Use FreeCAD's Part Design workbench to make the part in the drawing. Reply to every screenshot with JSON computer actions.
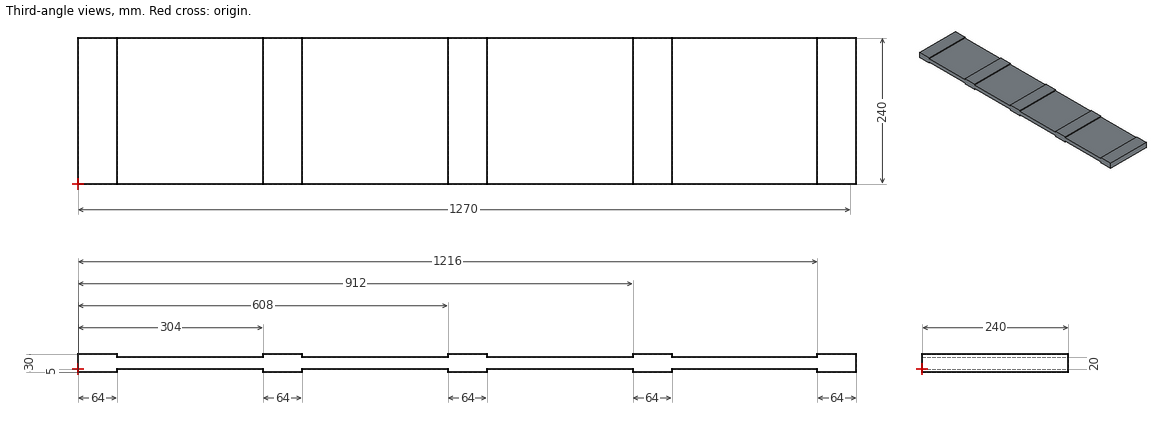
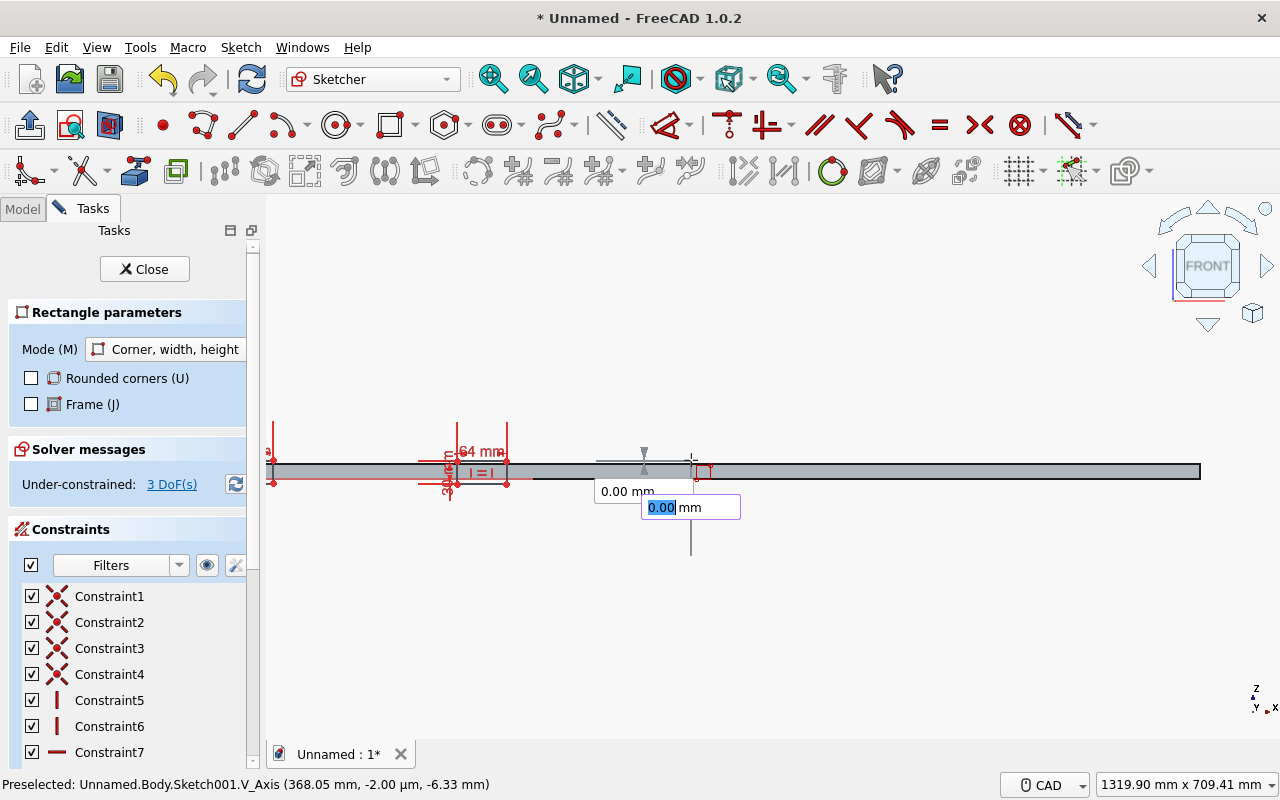
{"action": "scroll", "coordinate": [740, 483], "scroll_direction": "up", "scroll_amount": 8}
{"action": "mouse_move", "coordinate": [739, 482]}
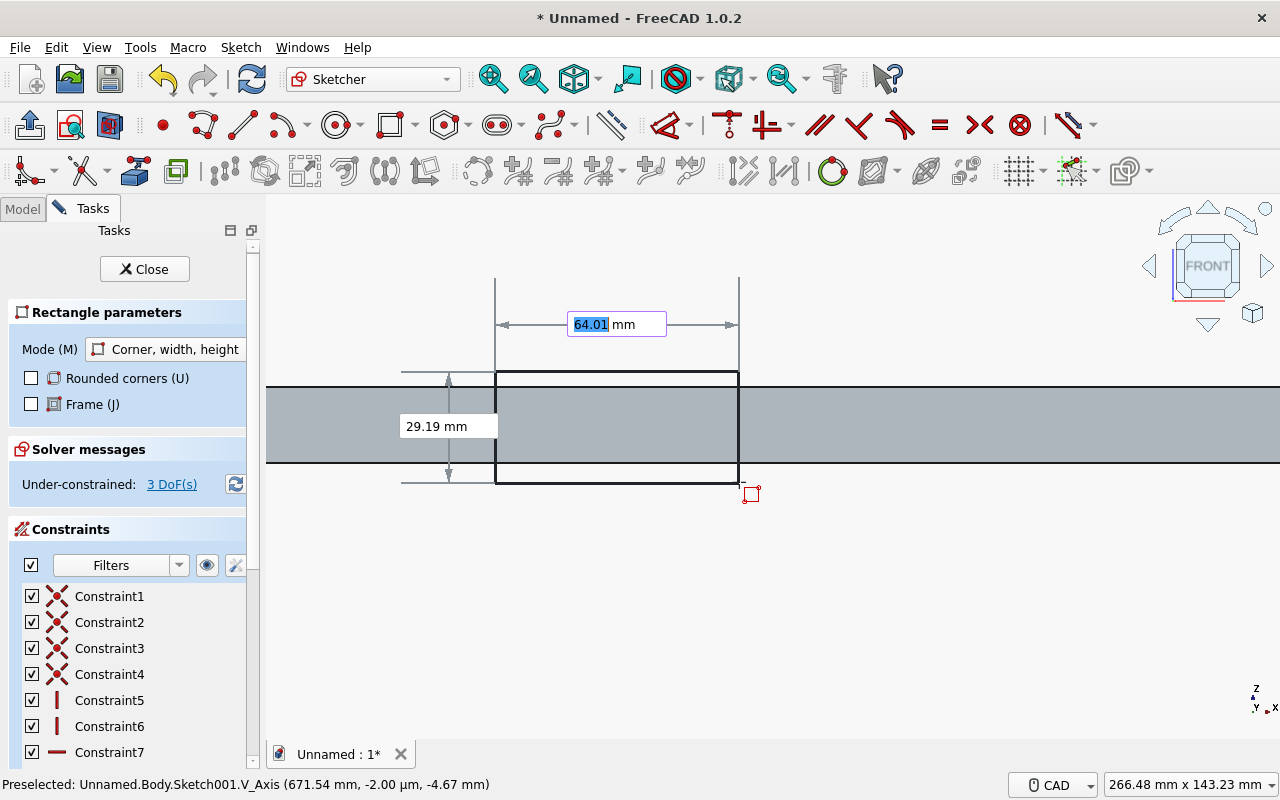
{"action": "type", "text": "64"}
{"action": "key", "text": "Tab"}
{"action": "type", "text": "30"}
{"action": "key", "text": "Return"}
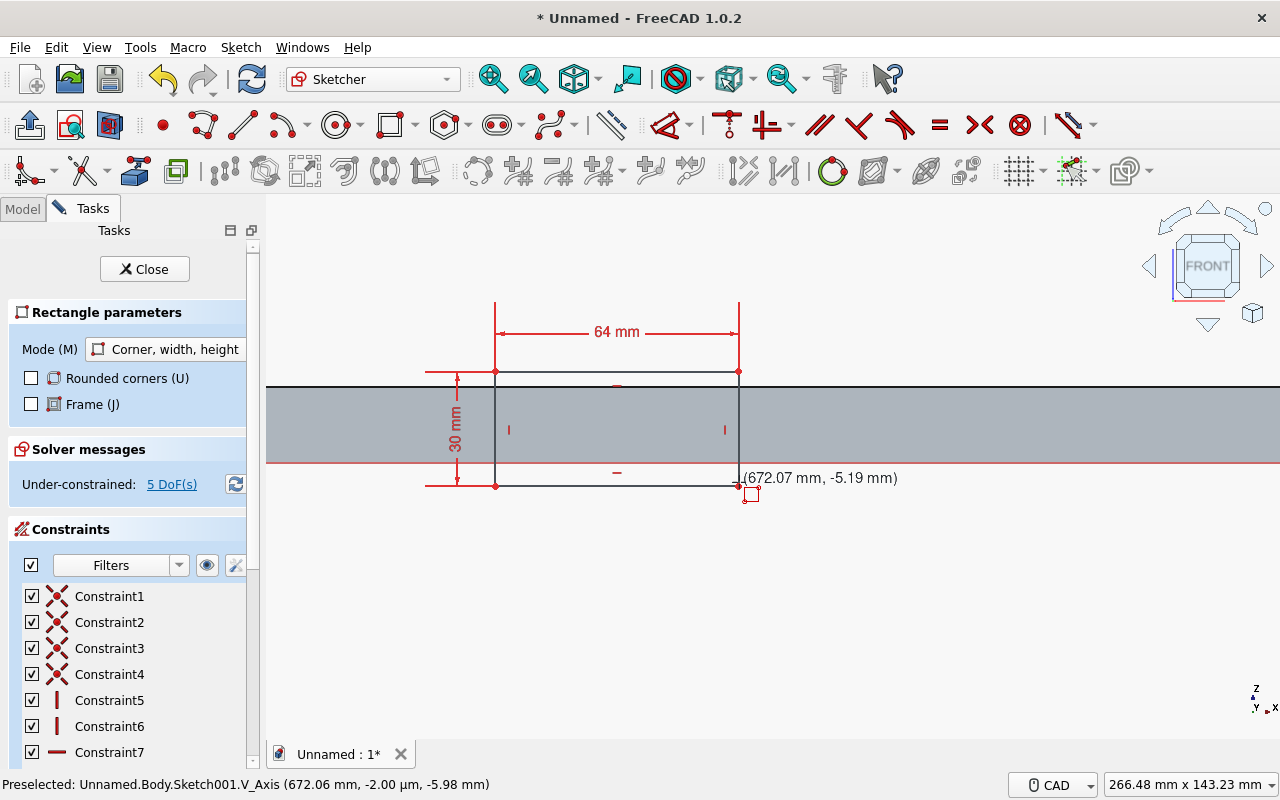
{"action": "scroll", "coordinate": [715, 472], "scroll_direction": "down", "scroll_amount": 11}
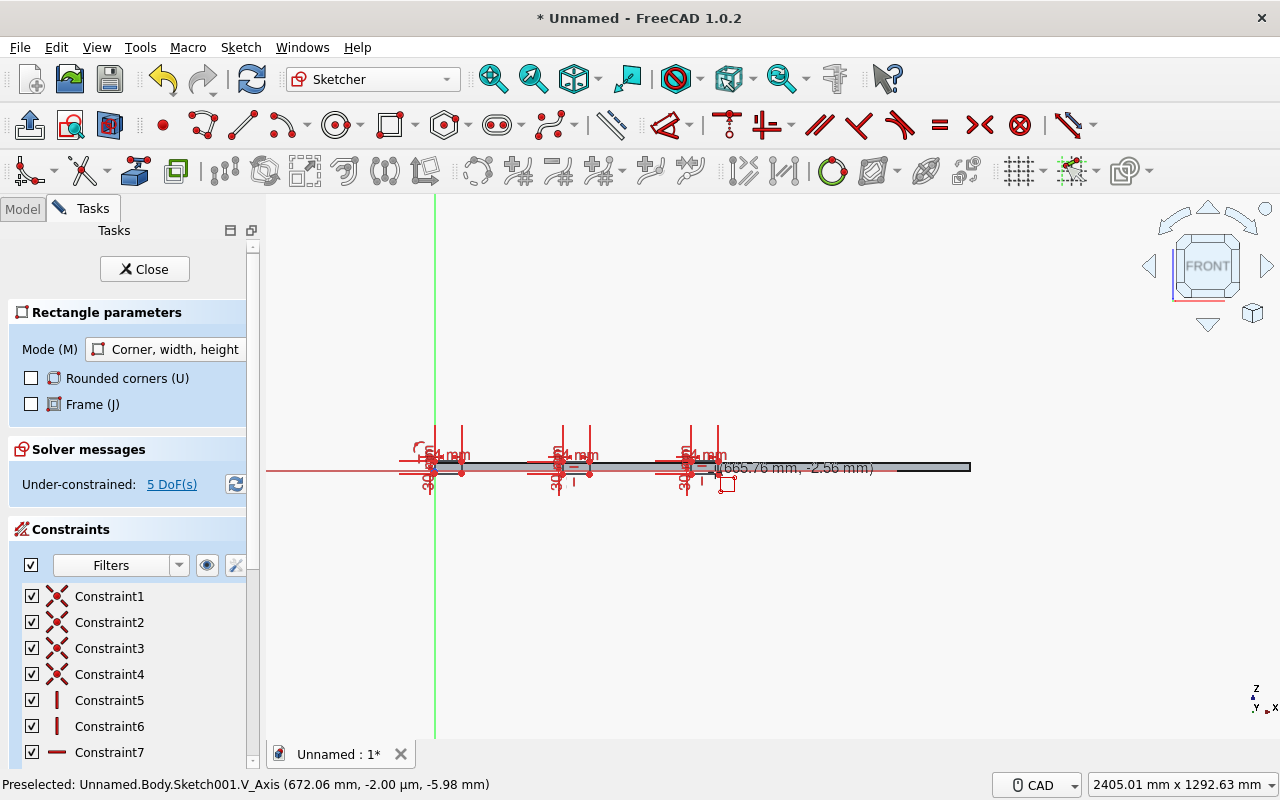
{"action": "scroll", "coordinate": [819, 461], "scroll_direction": "up", "scroll_amount": 3}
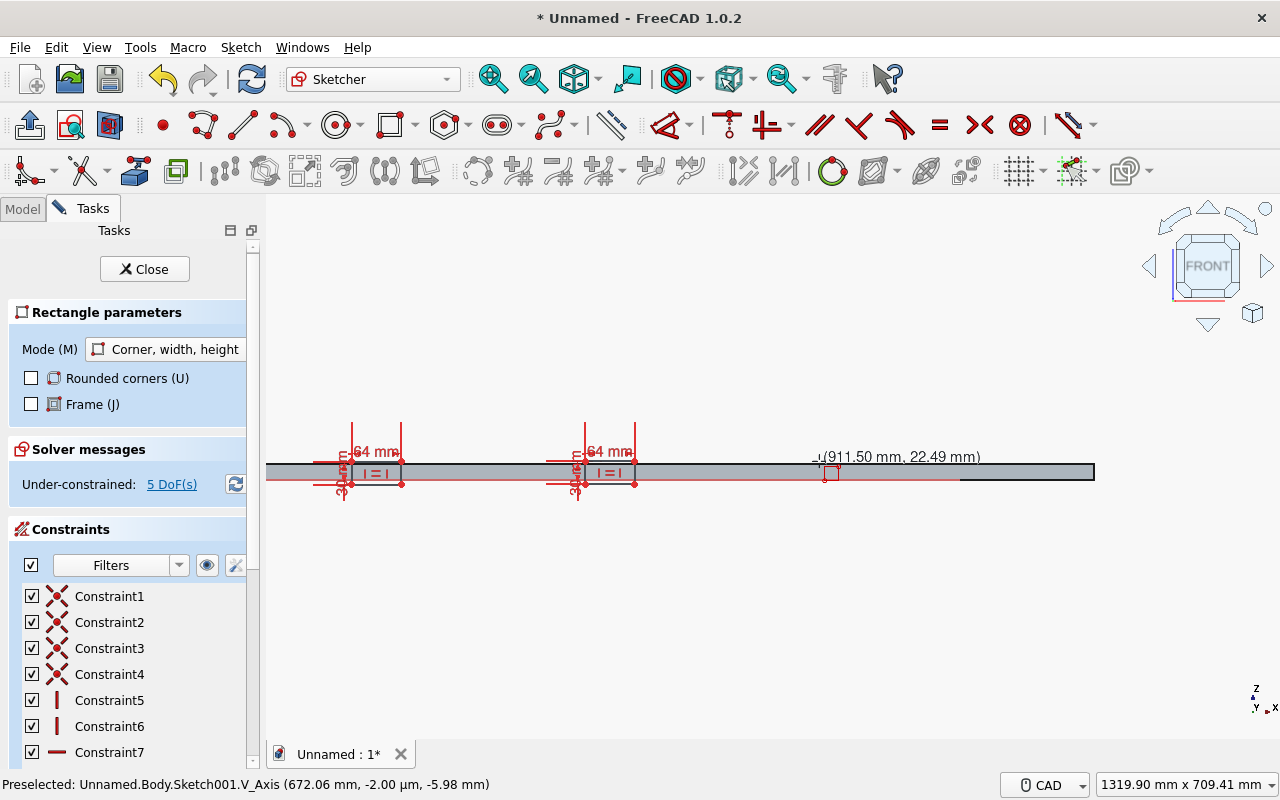
{"action": "left_click", "coordinate": [819, 460]}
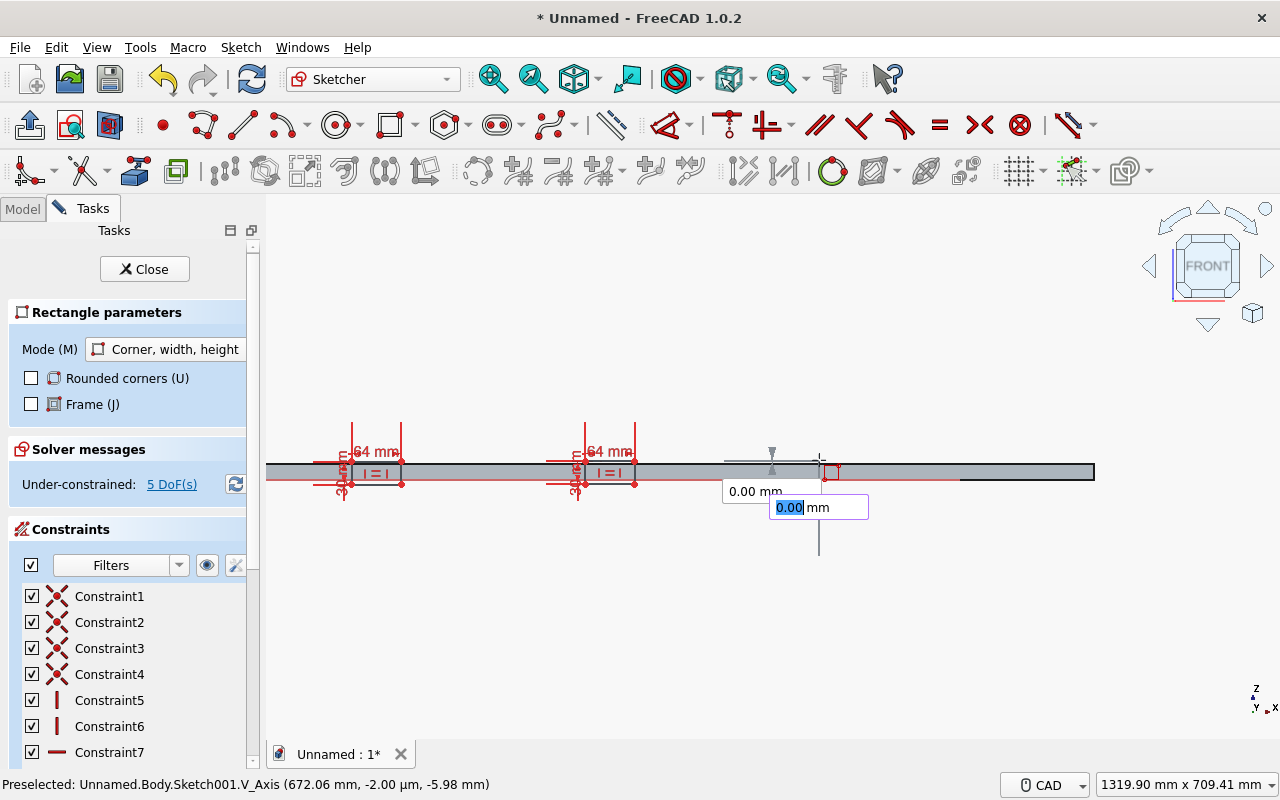
{"action": "scroll", "coordinate": [868, 484], "scroll_direction": "up", "scroll_amount": 8}
{"action": "mouse_move", "coordinate": [866, 480]}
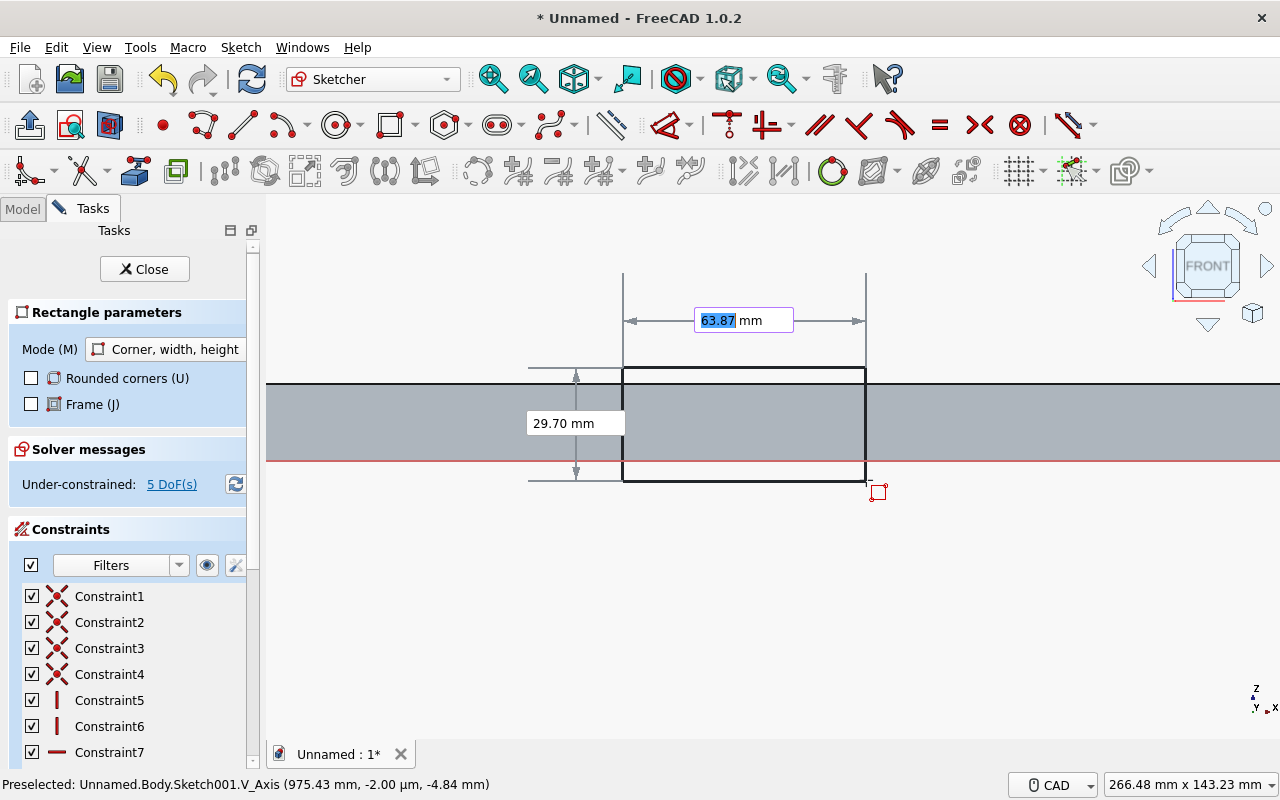
{"action": "type", "text": "64"}
{"action": "key", "text": "Tab"}
{"action": "type", "text": "30"}
{"action": "key", "text": "Return"}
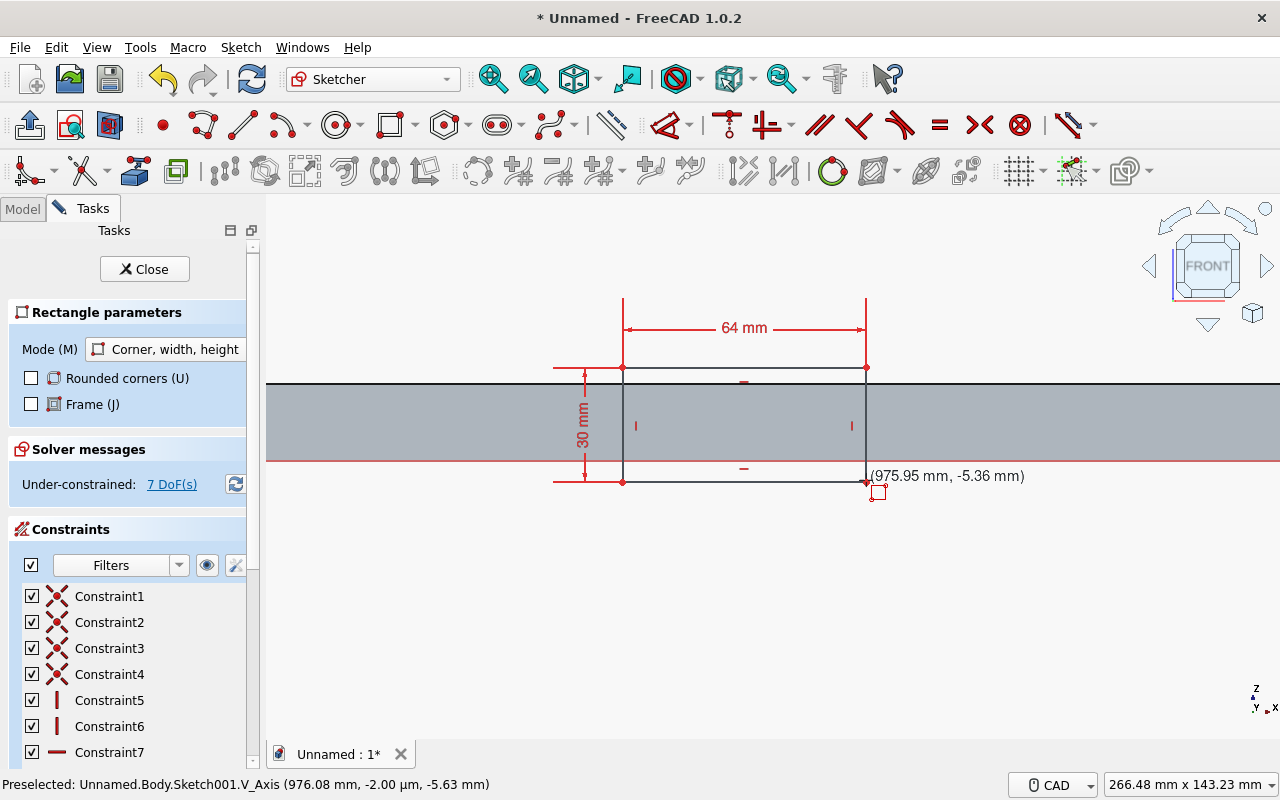
{"action": "scroll", "coordinate": [844, 472], "scroll_direction": "down", "scroll_amount": 11}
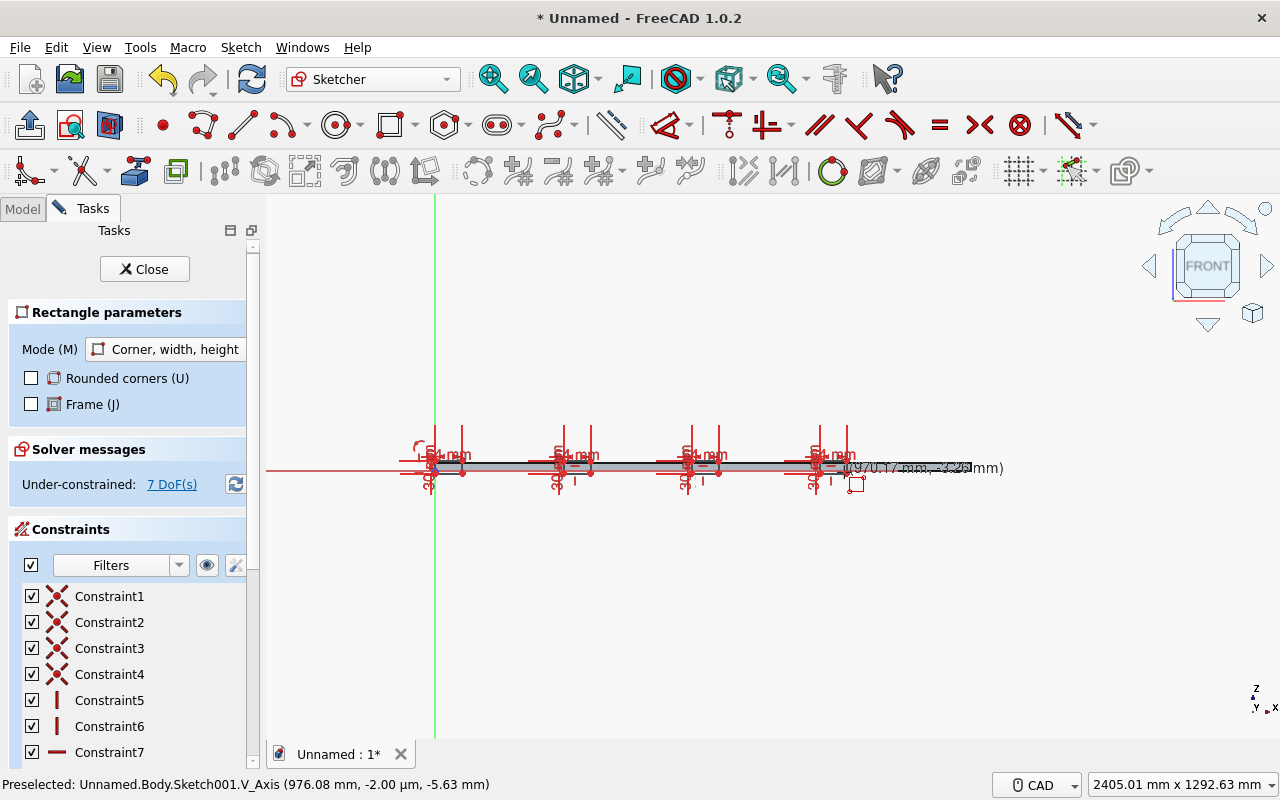
{"action": "scroll", "coordinate": [948, 461], "scroll_direction": "up", "scroll_amount": 3}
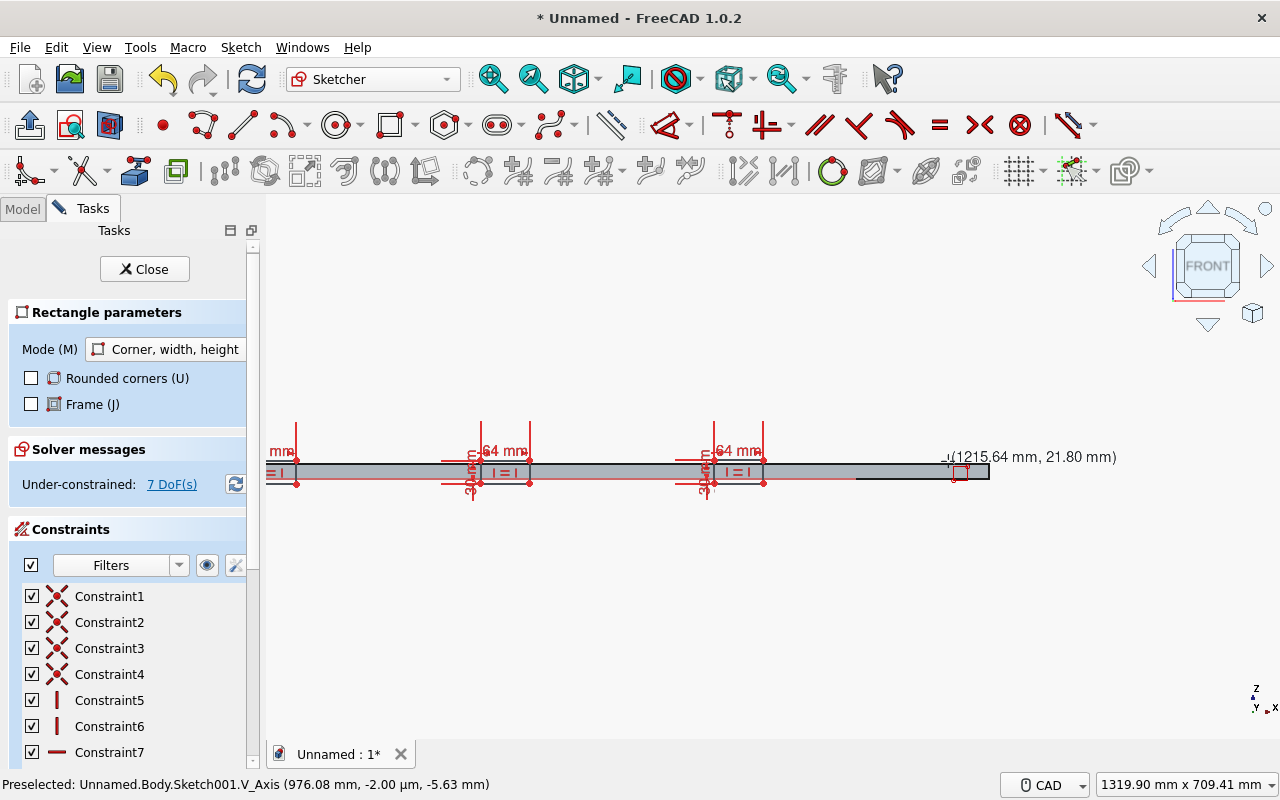
{"action": "left_click", "coordinate": [948, 460]}